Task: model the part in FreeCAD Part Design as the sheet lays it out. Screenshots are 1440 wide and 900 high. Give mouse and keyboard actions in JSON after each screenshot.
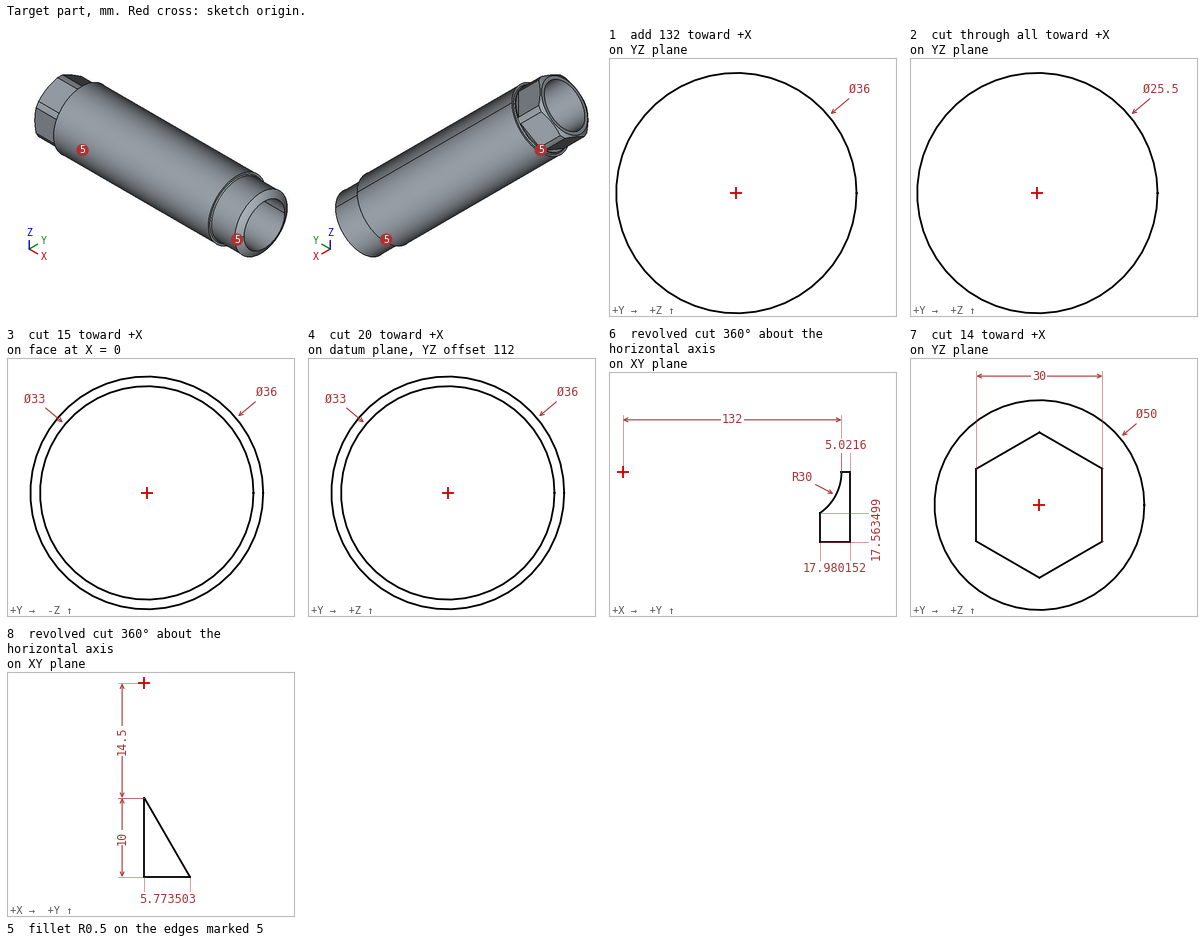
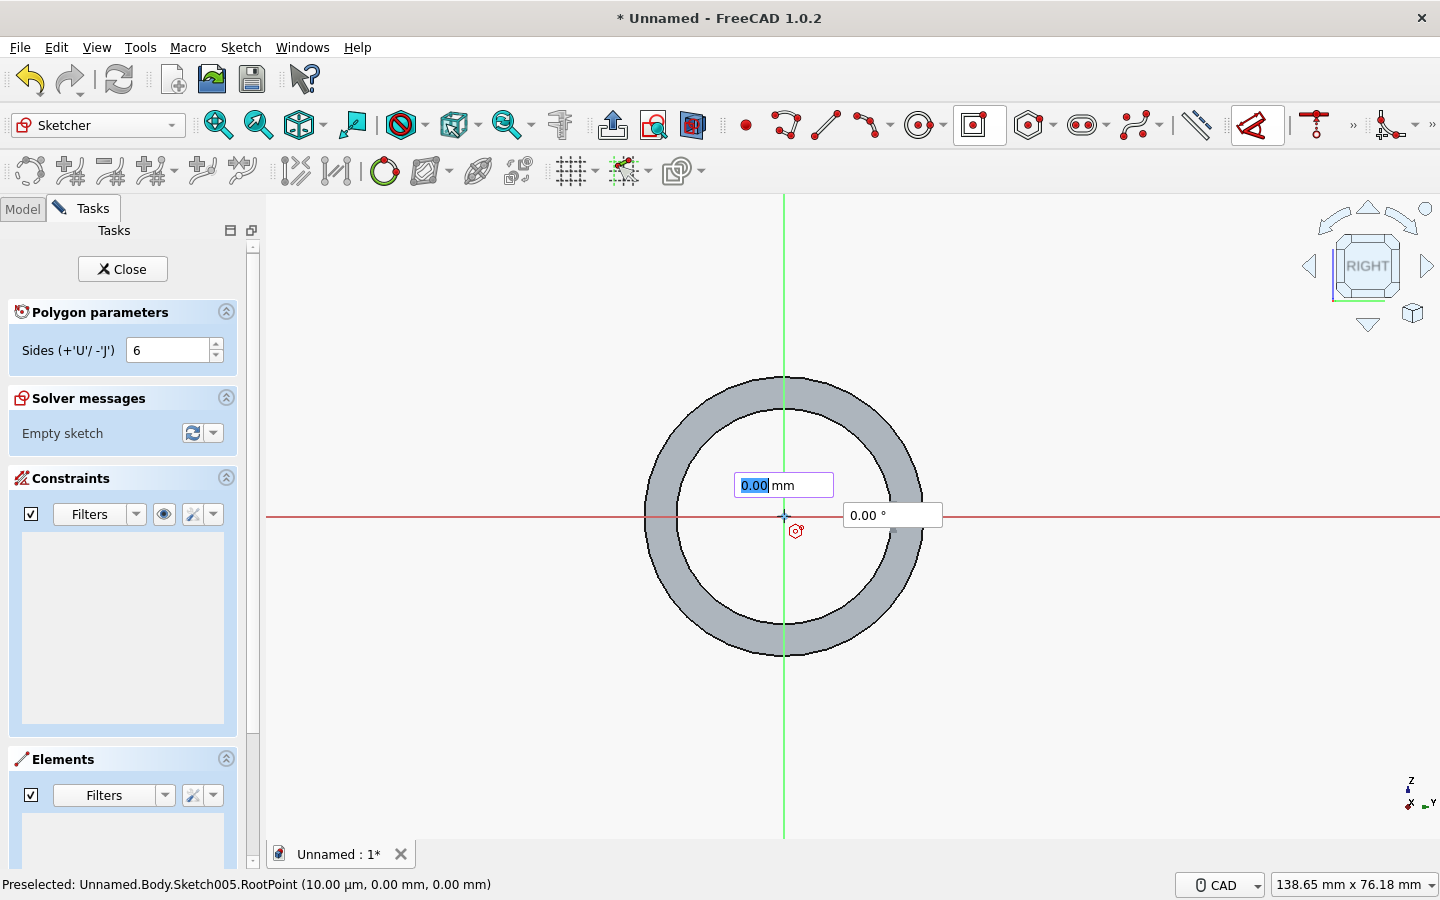
{"action": "left_click", "coordinate": [784, 663]}
{"action": "right_click", "coordinate": [784, 663]}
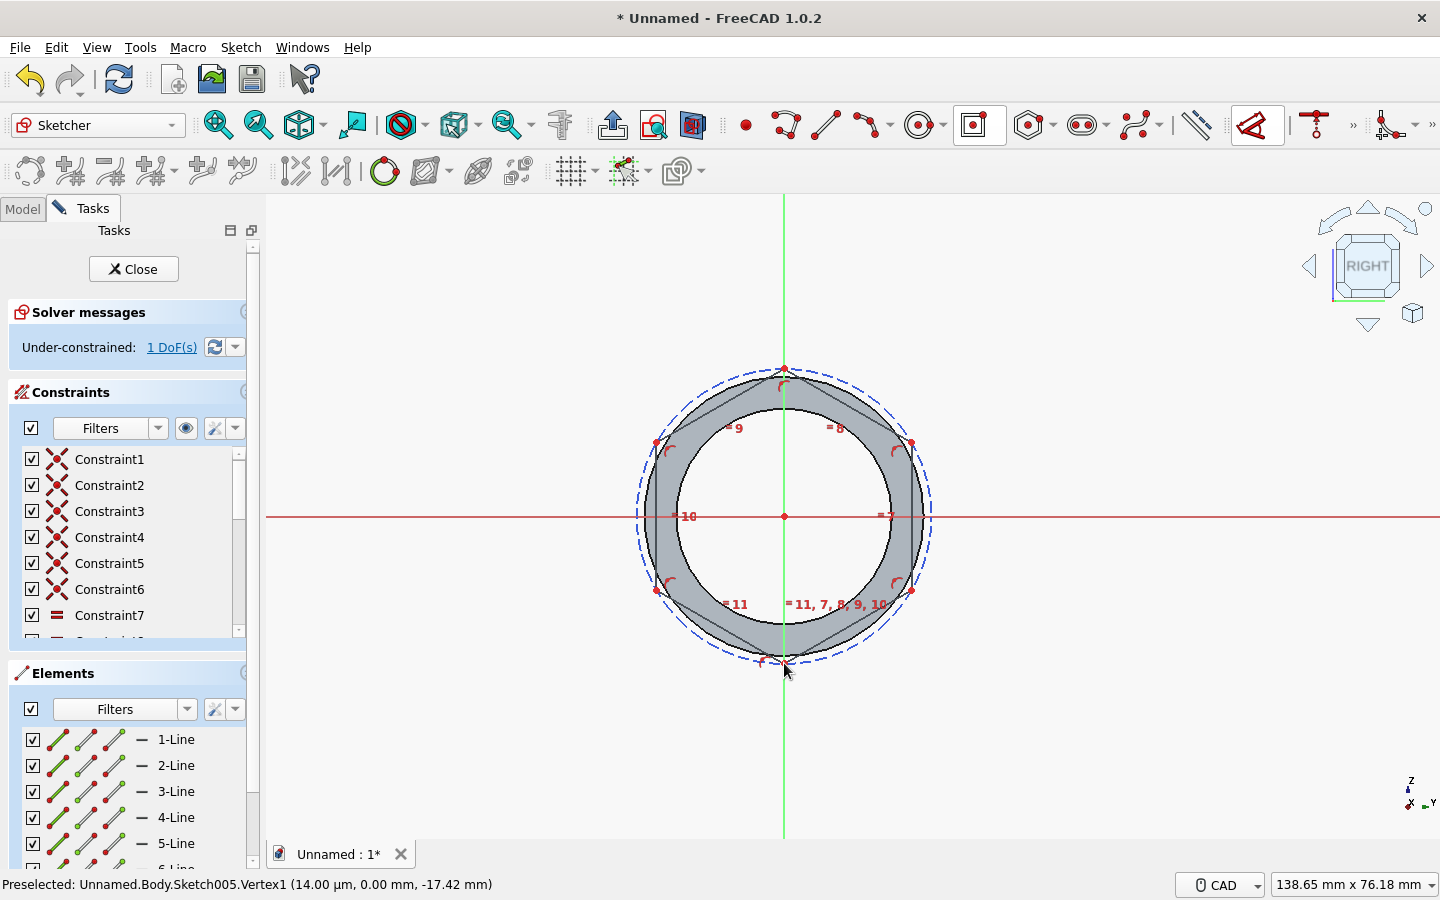
{"action": "left_click", "coordinate": [920, 126]}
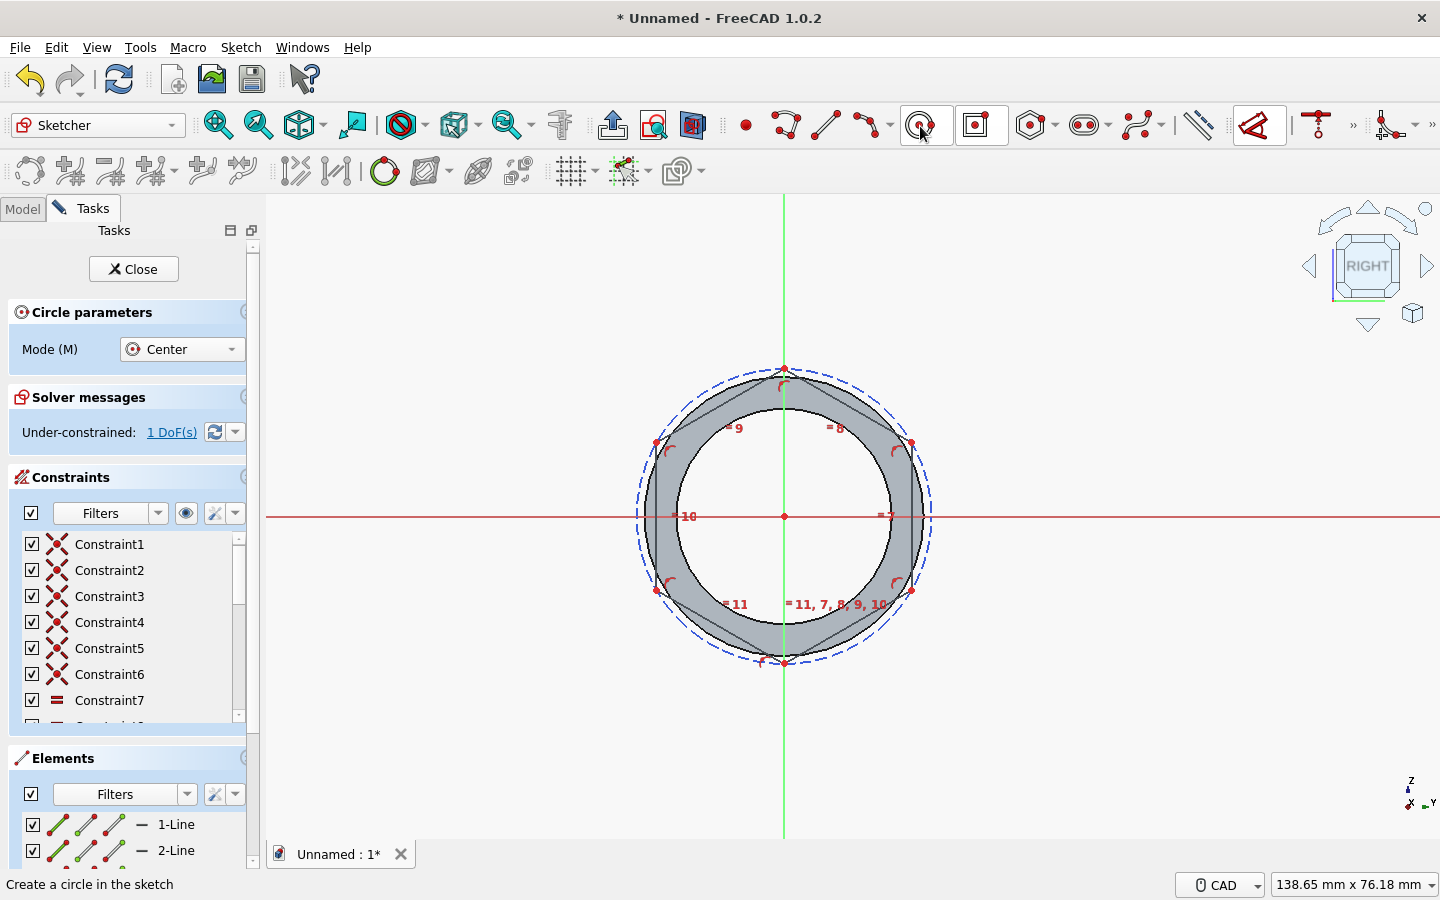
{"action": "left_click", "coordinate": [784, 516]}
{"action": "mouse_move", "coordinate": [934, 367]}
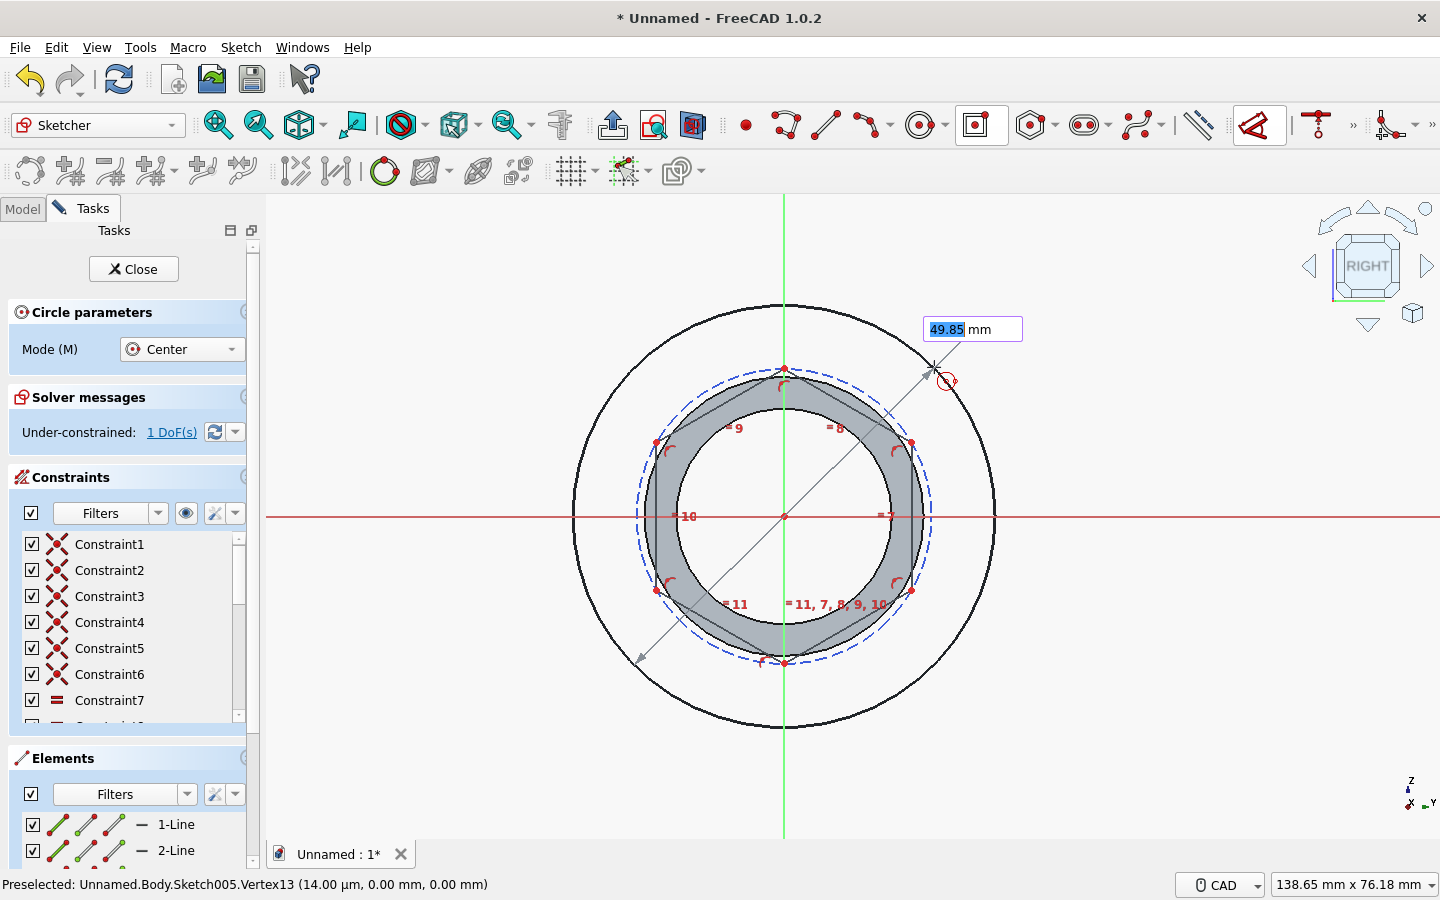
{"action": "type", "text": "50"}
{"action": "key", "text": "Return"}
{"action": "key", "text": "Escape"}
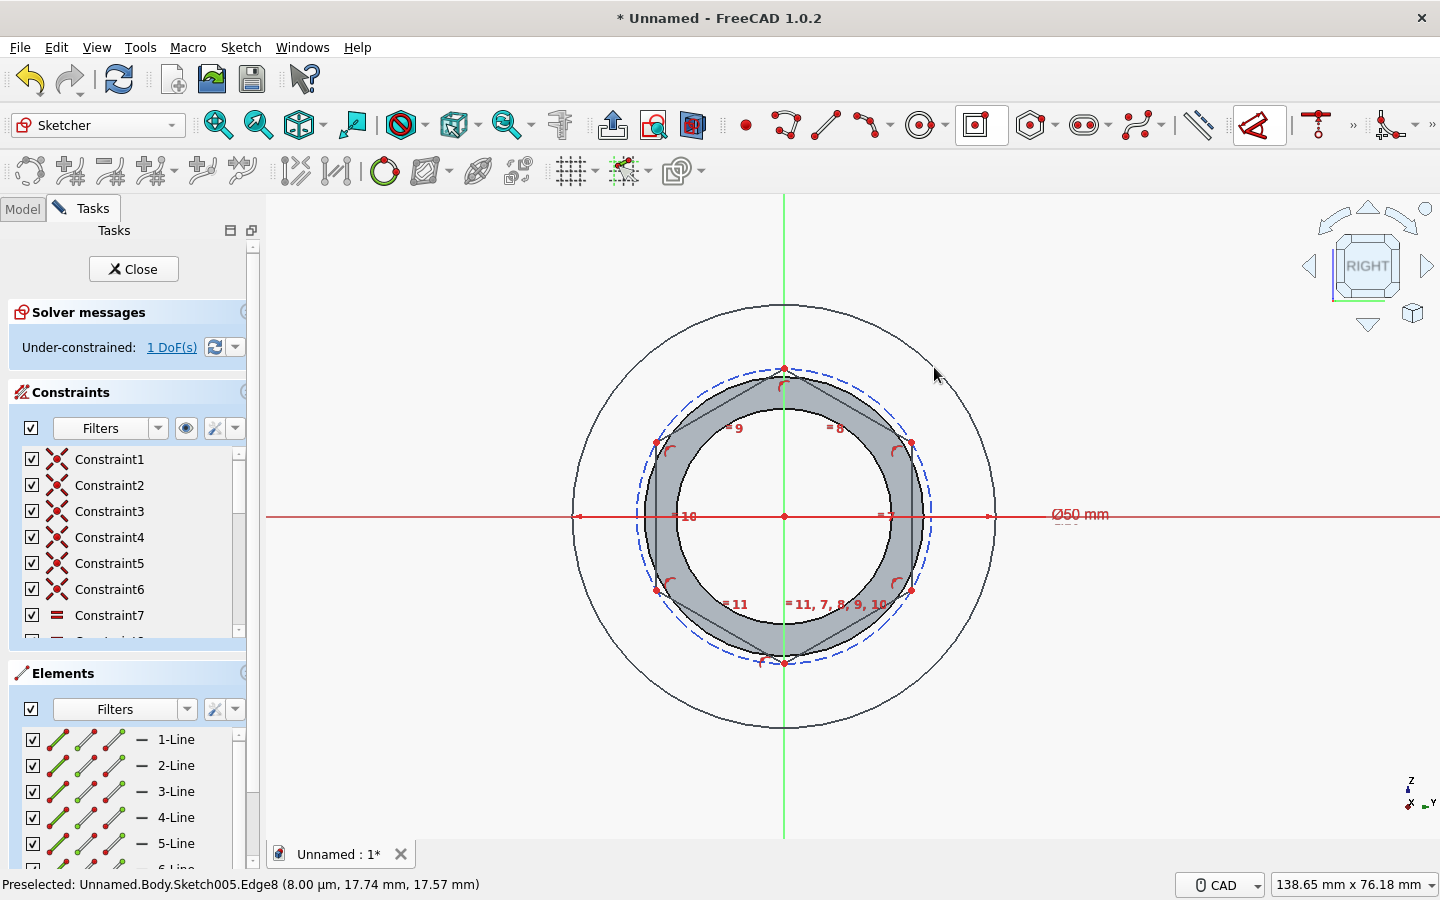
{"action": "left_click", "coordinate": [656, 443]}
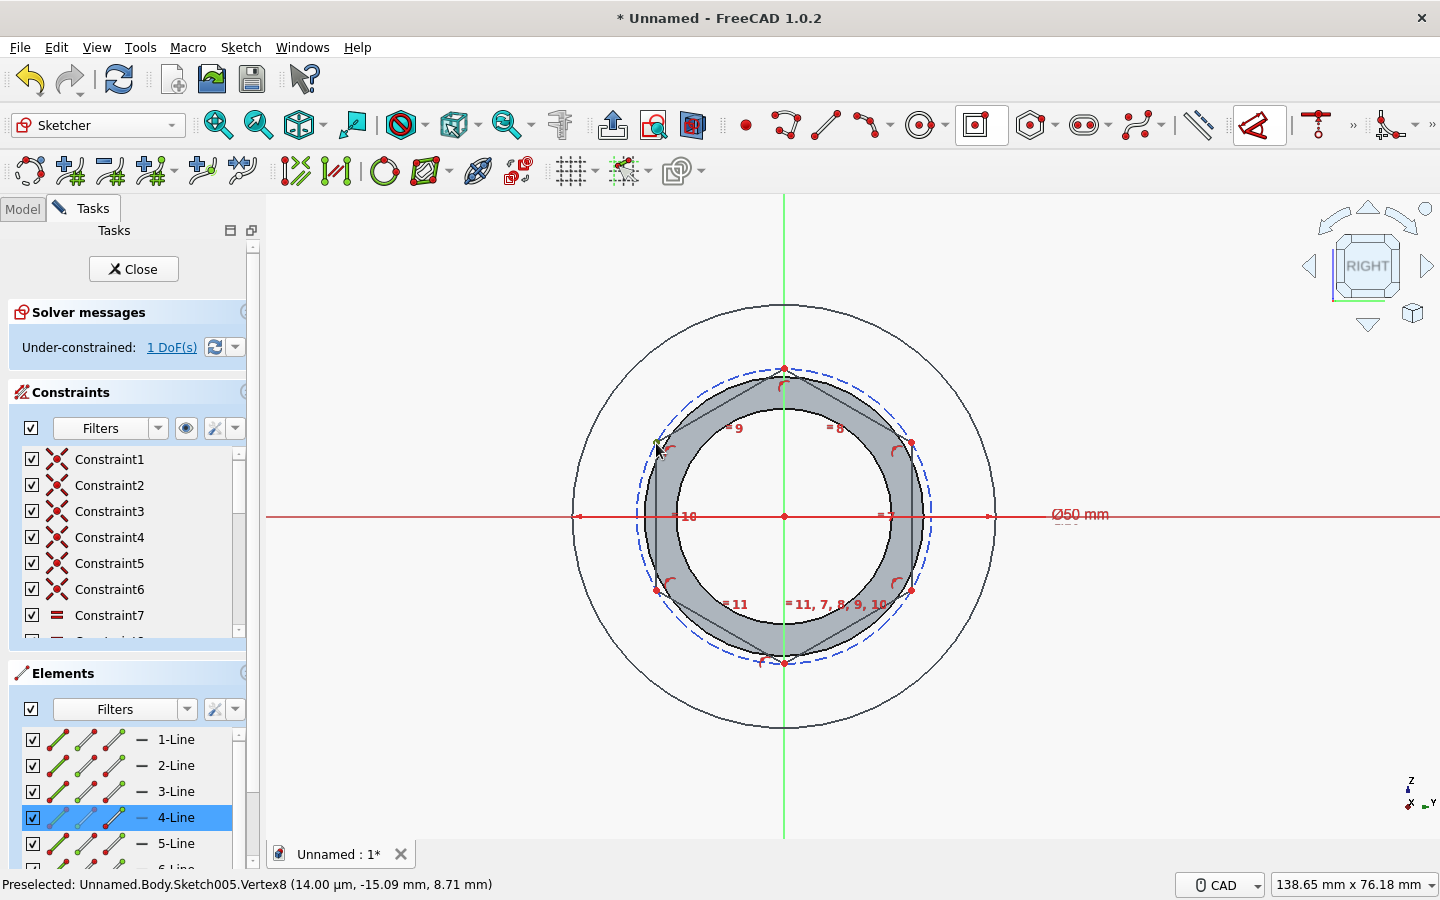
{"action": "left_click", "coordinate": [912, 590]}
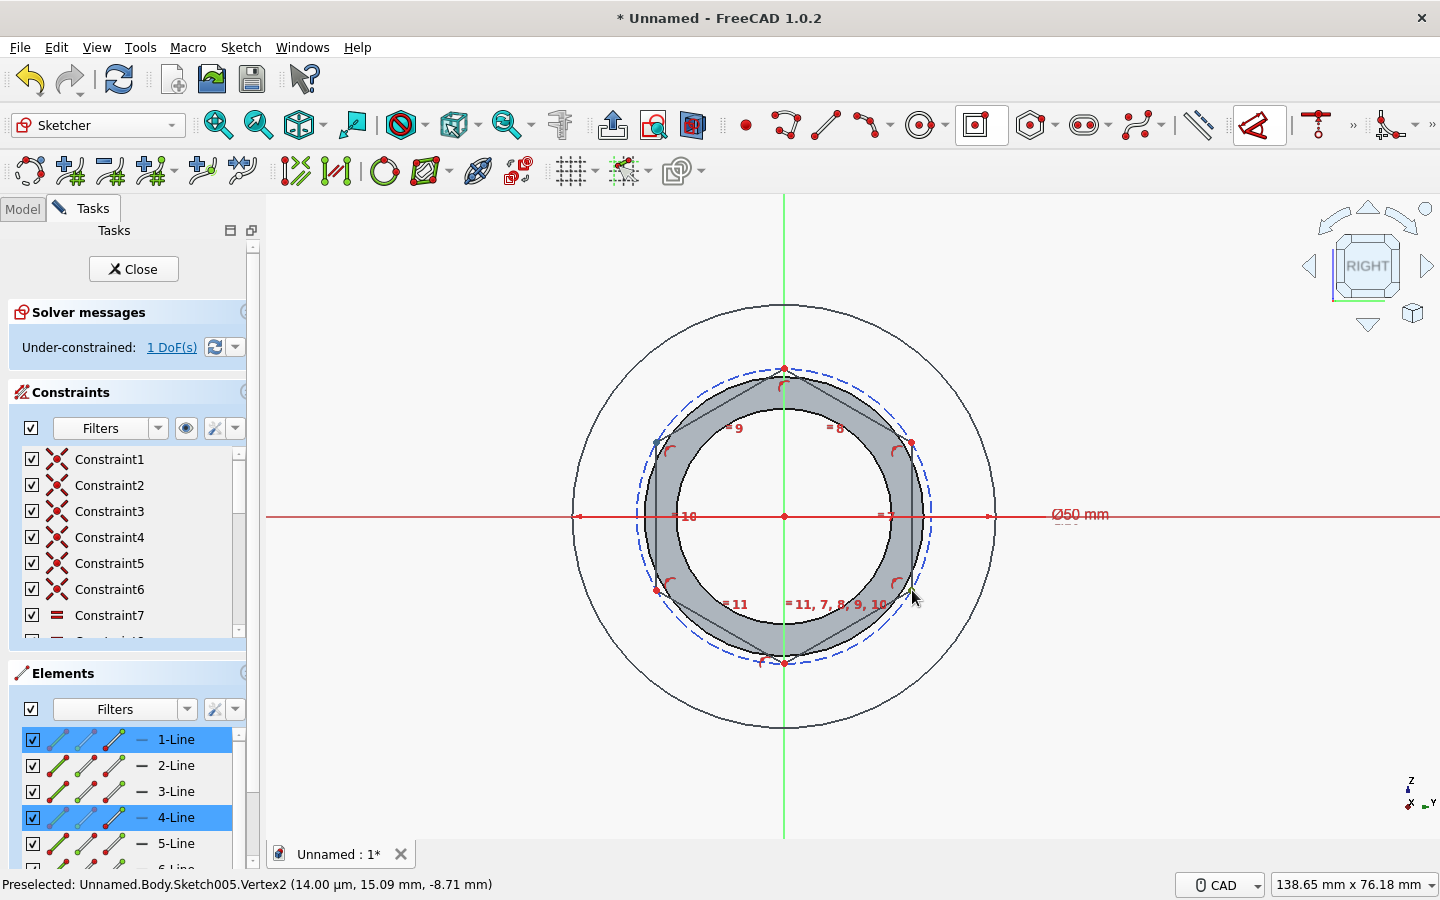
{"action": "key", "text": "l"}